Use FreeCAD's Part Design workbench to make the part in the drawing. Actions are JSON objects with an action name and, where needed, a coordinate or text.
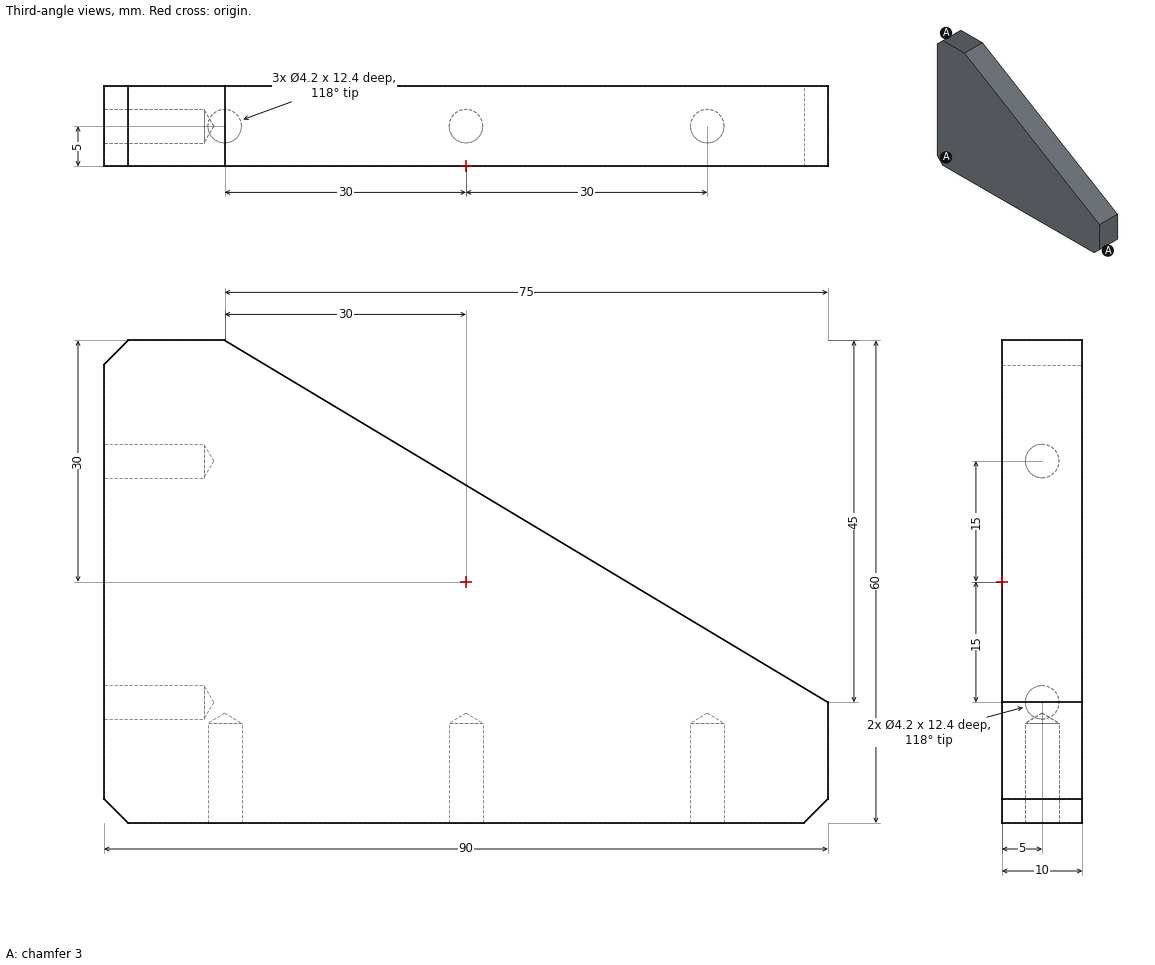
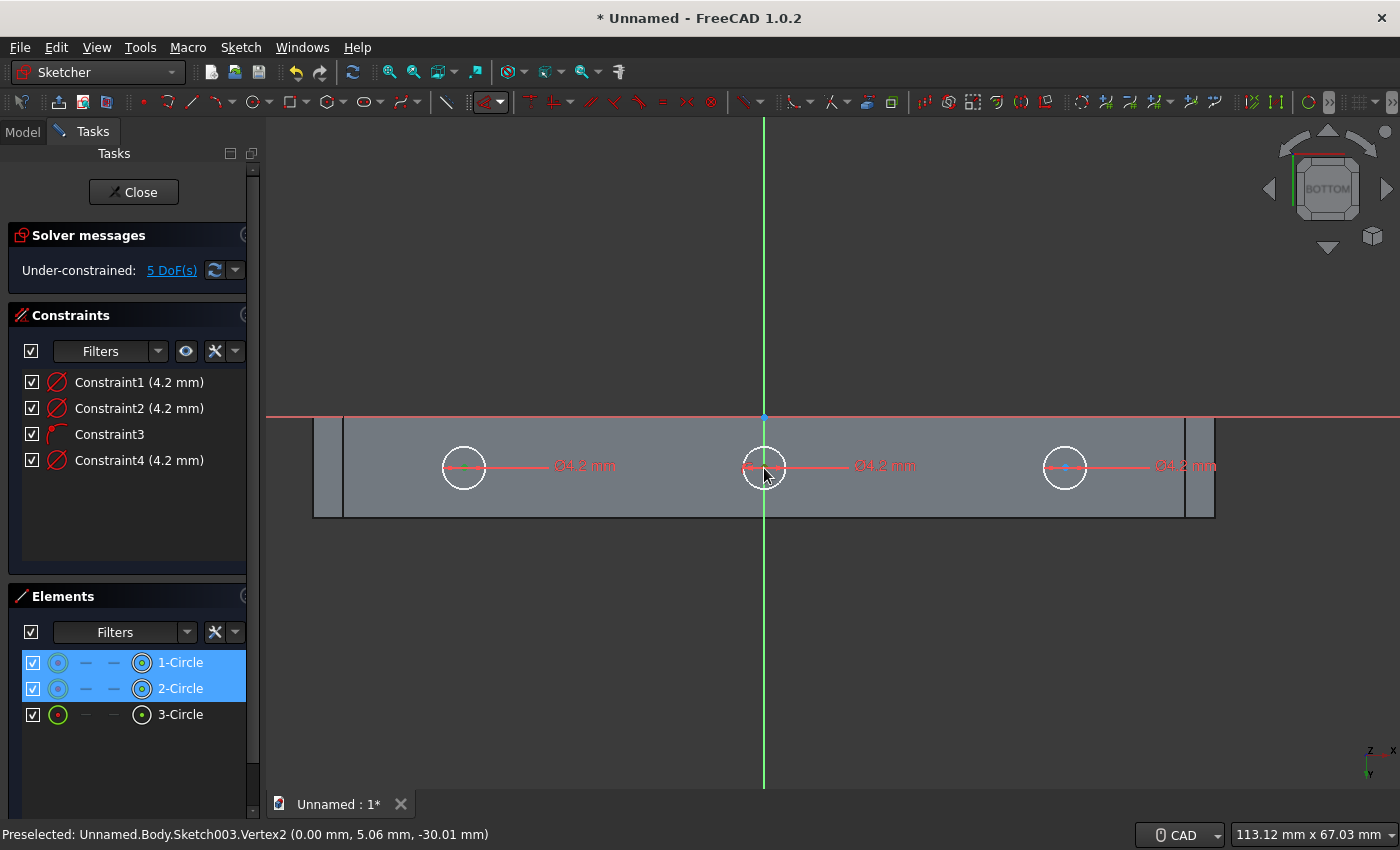
{"action": "key", "text": "h"}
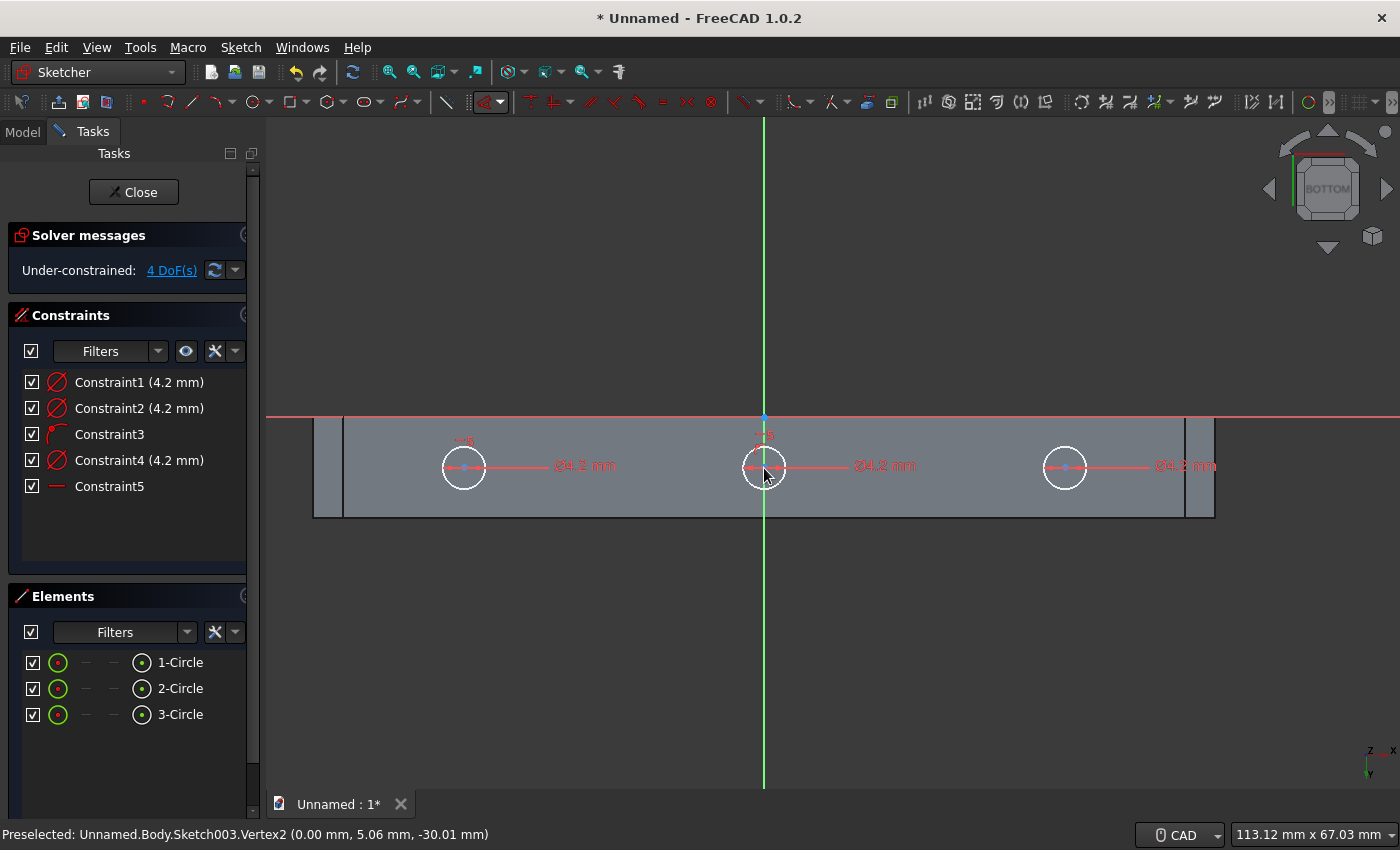
{"action": "left_click", "coordinate": [764, 468]}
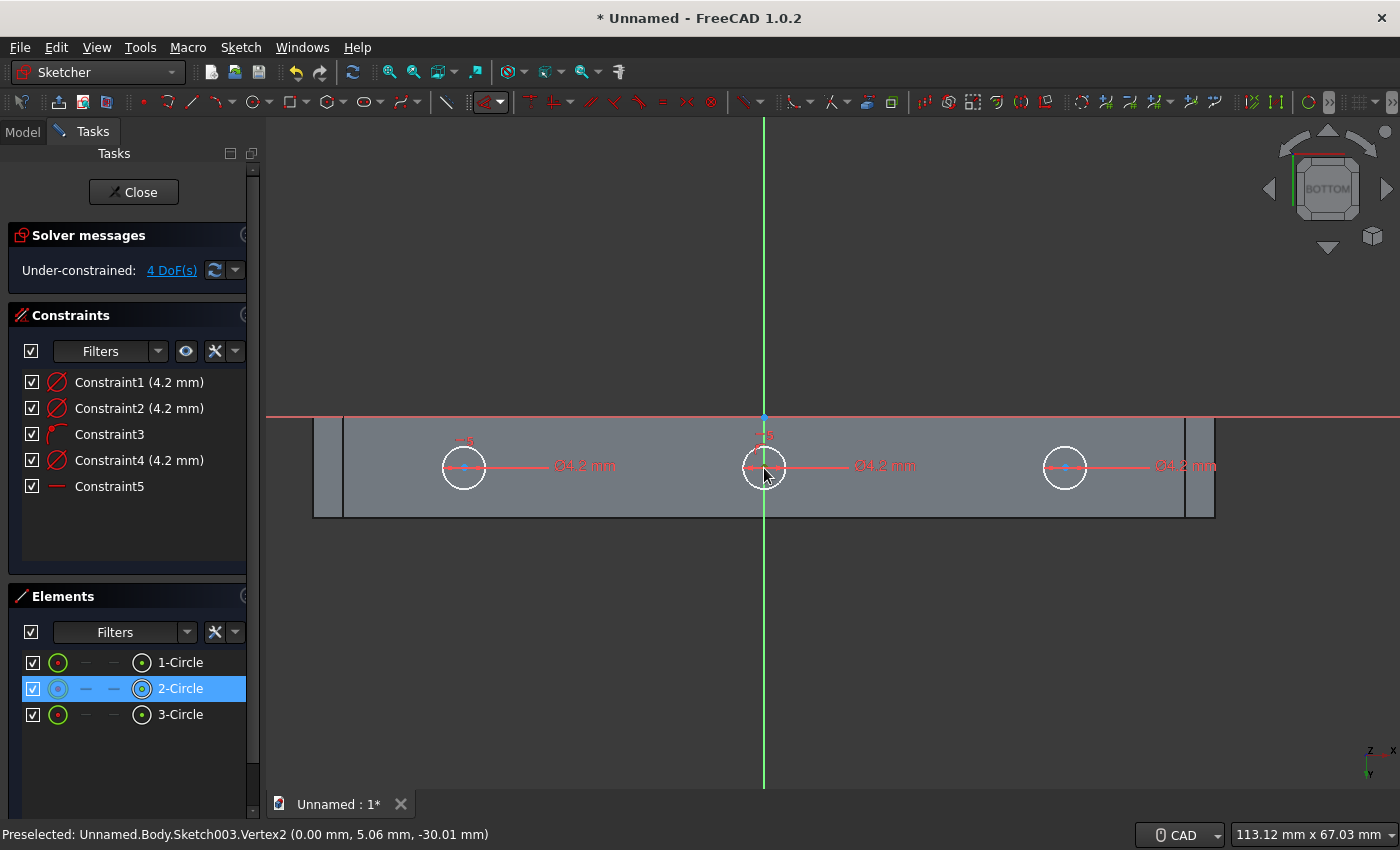
{"action": "left_click", "coordinate": [1065, 468]}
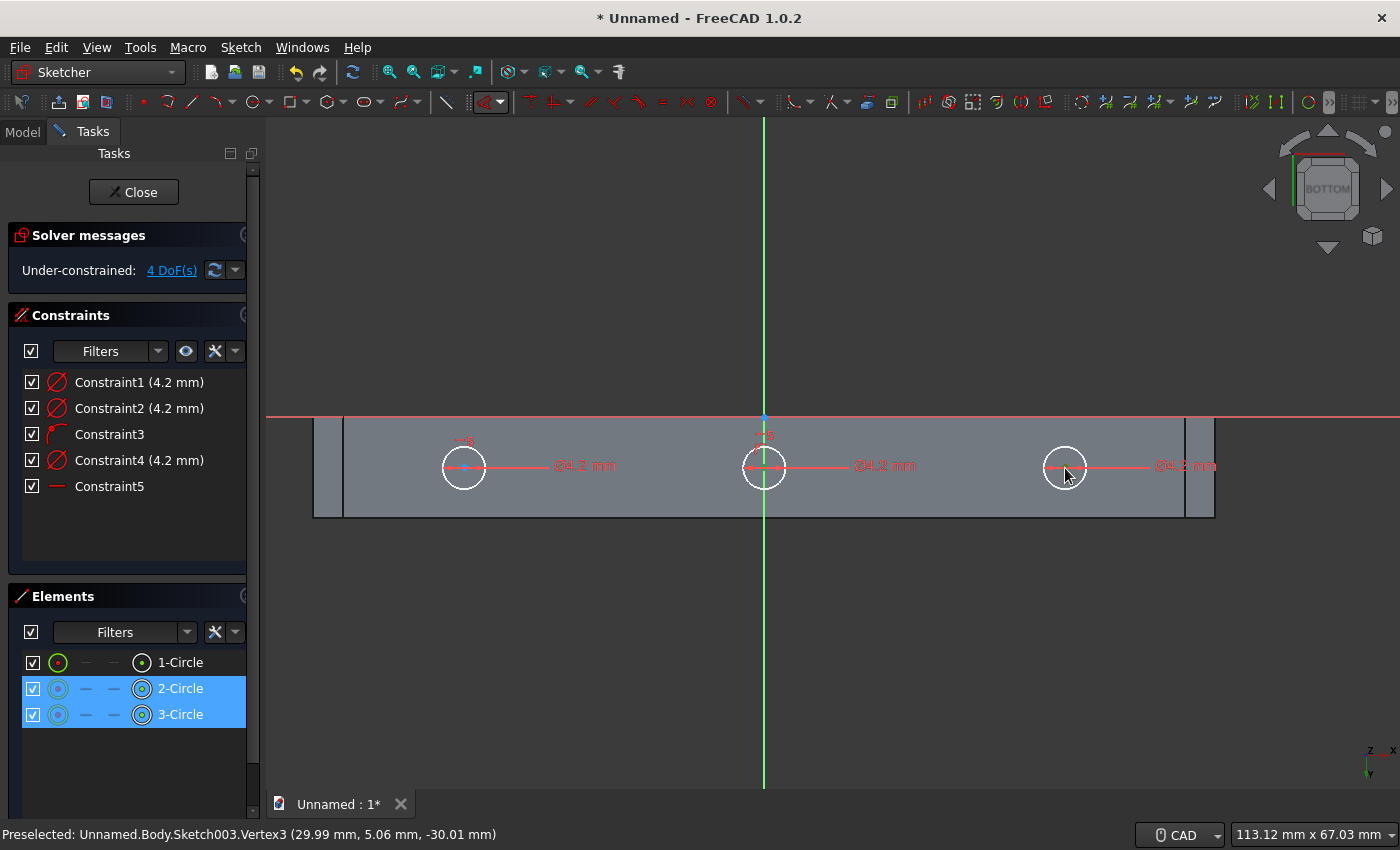
{"action": "key", "text": "h"}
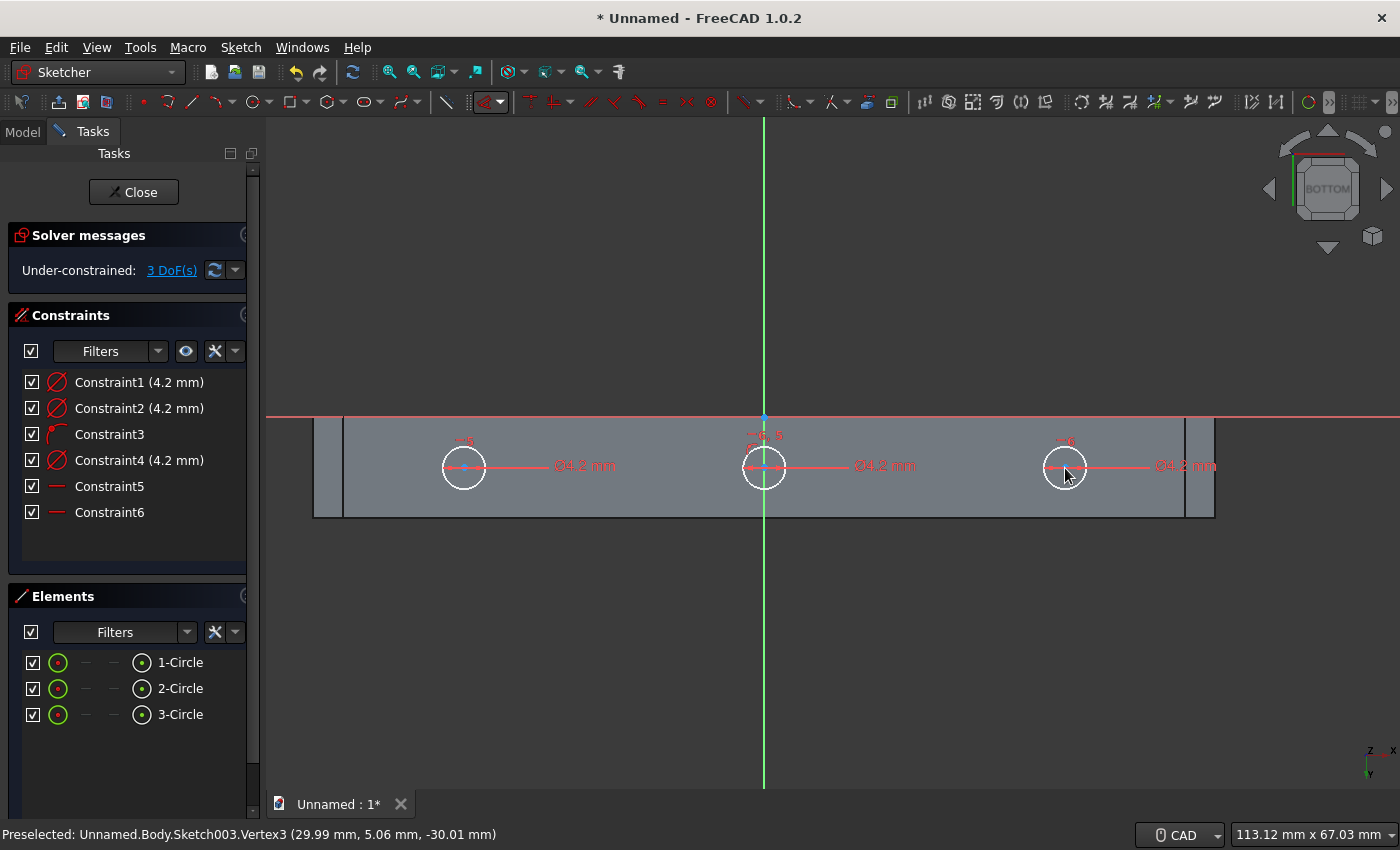
{"action": "key", "text": "d"}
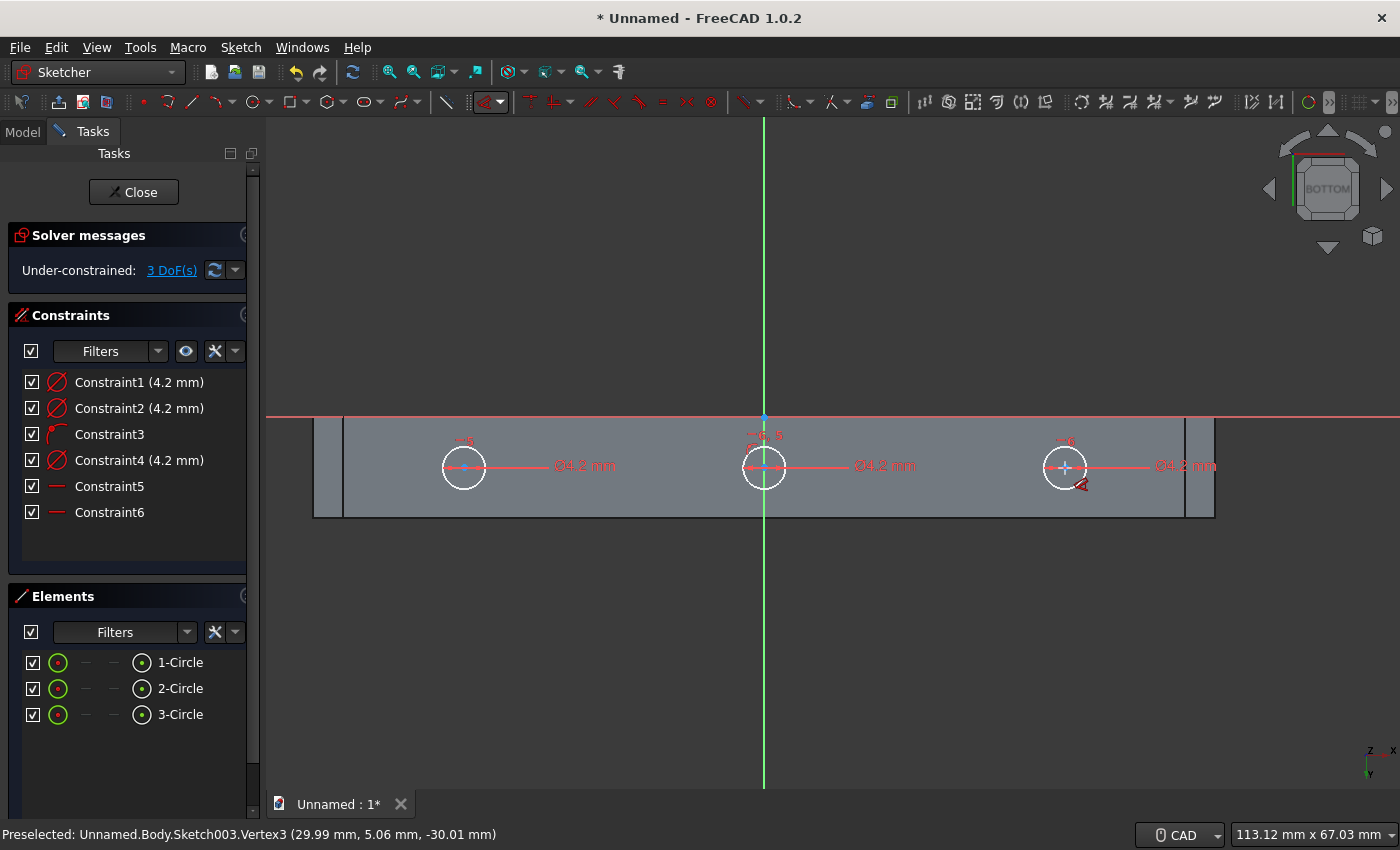
{"action": "left_click", "coordinate": [464, 468]}
{"action": "left_click", "coordinate": [430, 443]}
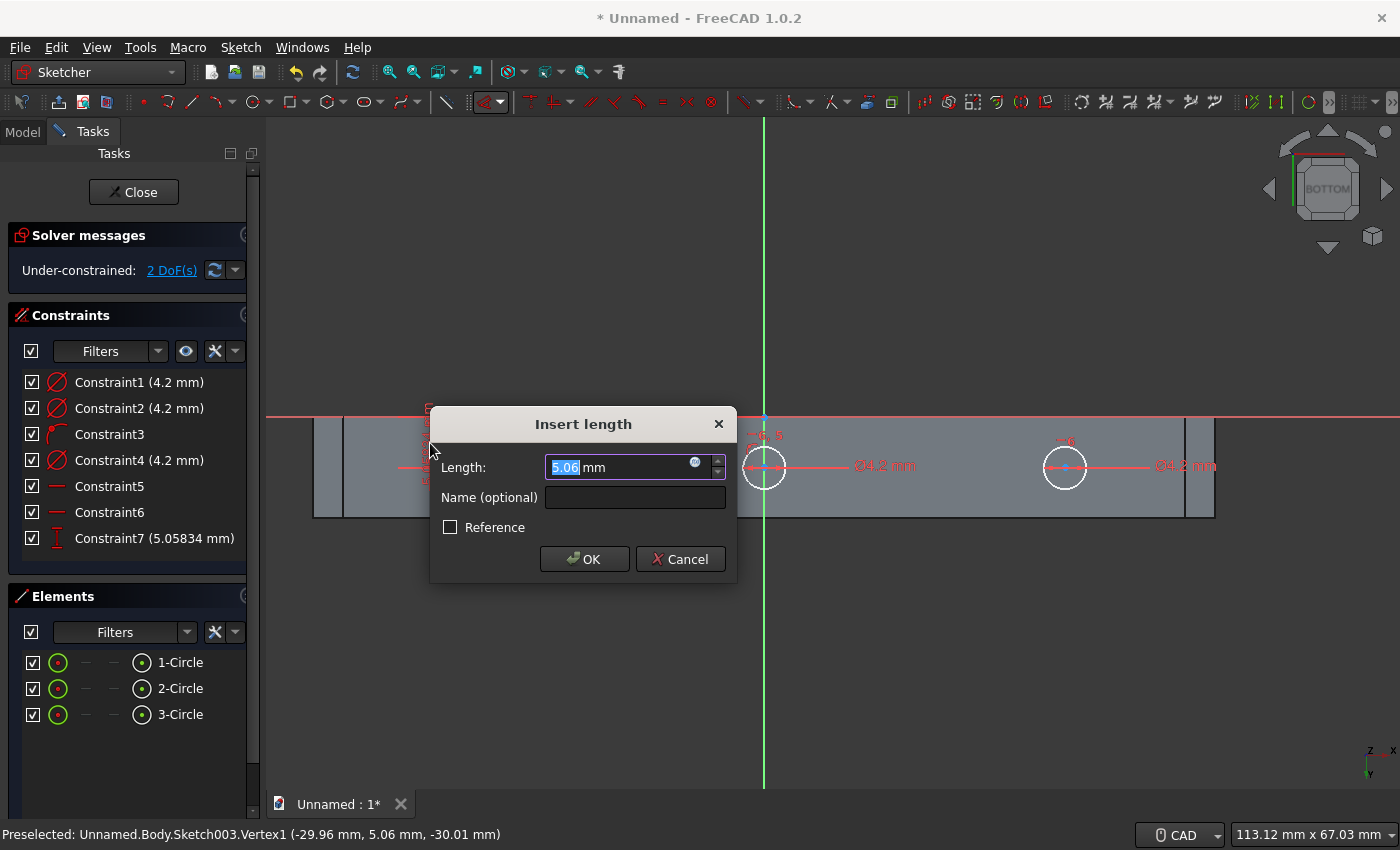
{"action": "type", "text": "5"}
{"action": "key", "text": "Return"}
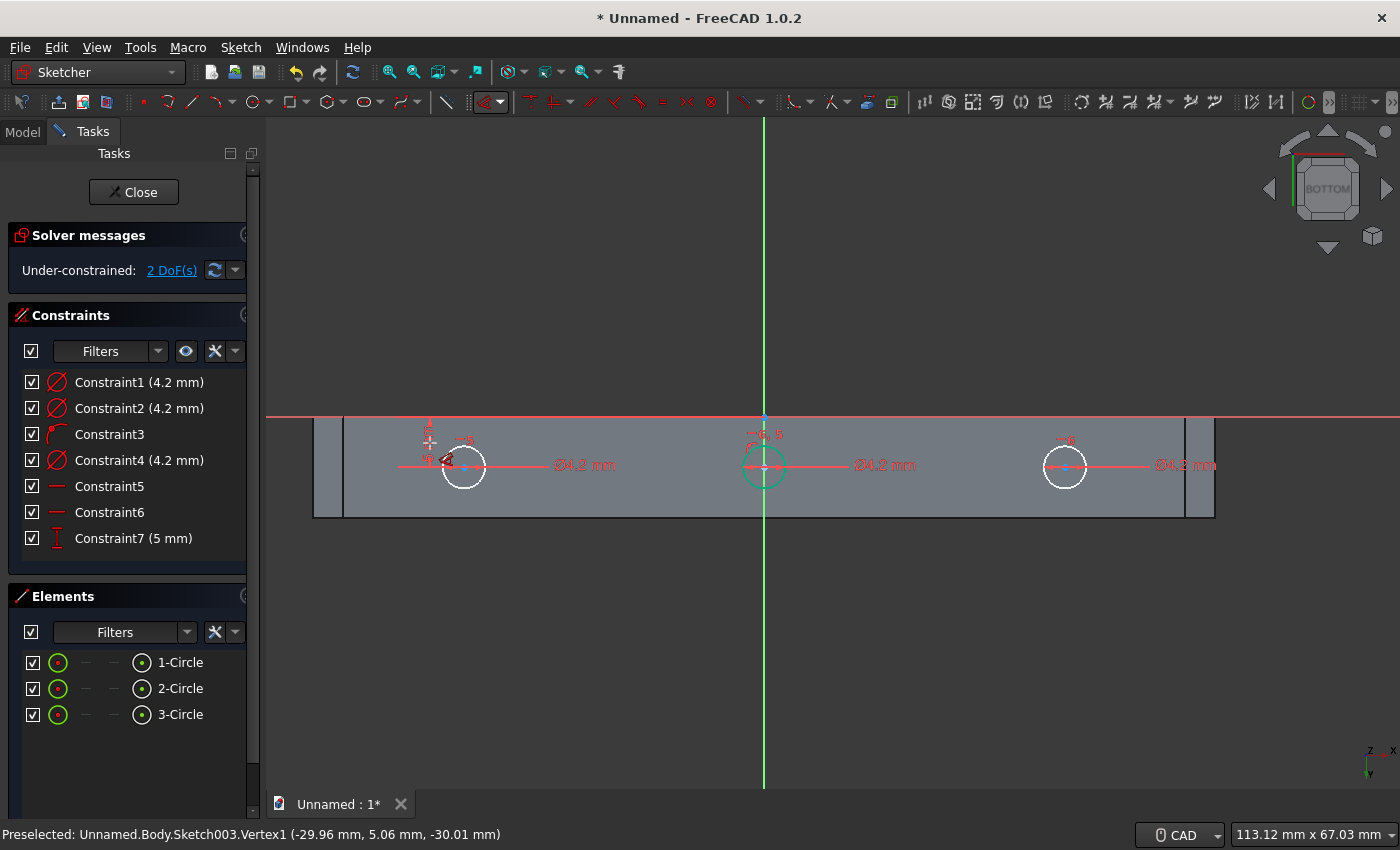
{"action": "left_click", "coordinate": [464, 467]}
{"action": "left_click", "coordinate": [614, 383]}